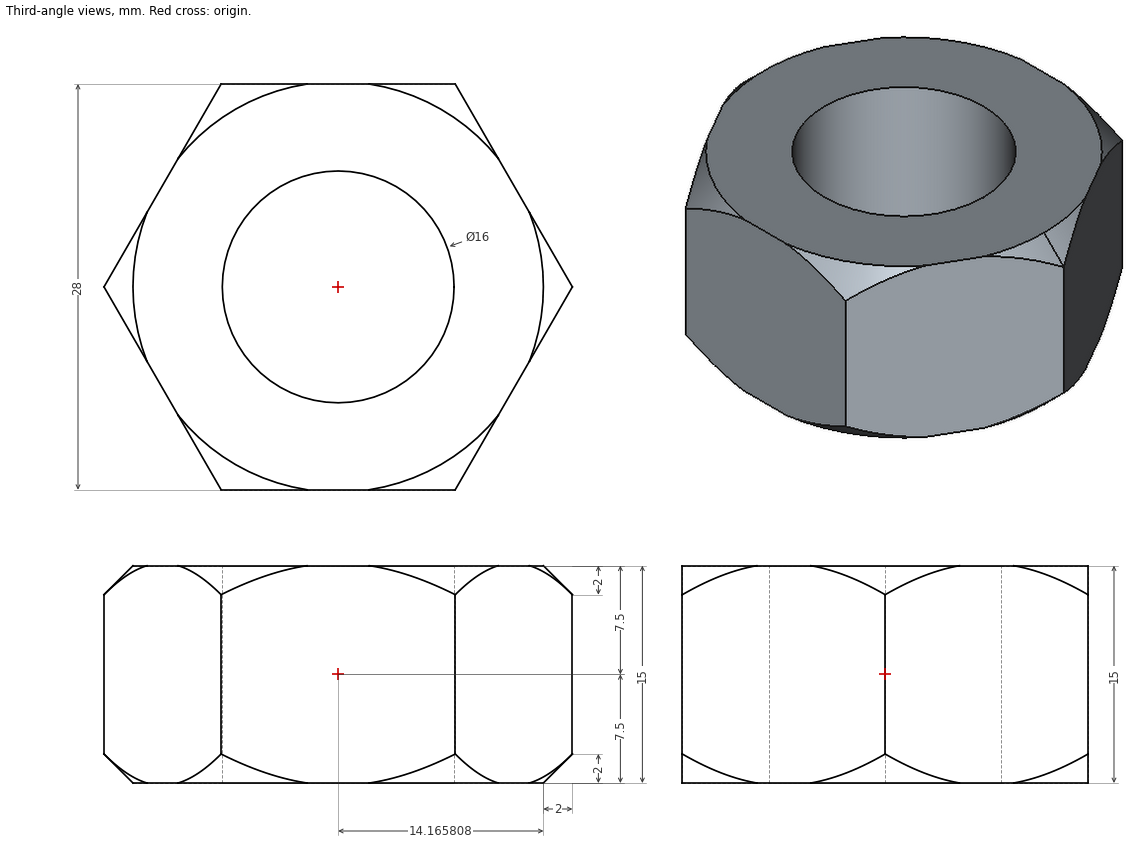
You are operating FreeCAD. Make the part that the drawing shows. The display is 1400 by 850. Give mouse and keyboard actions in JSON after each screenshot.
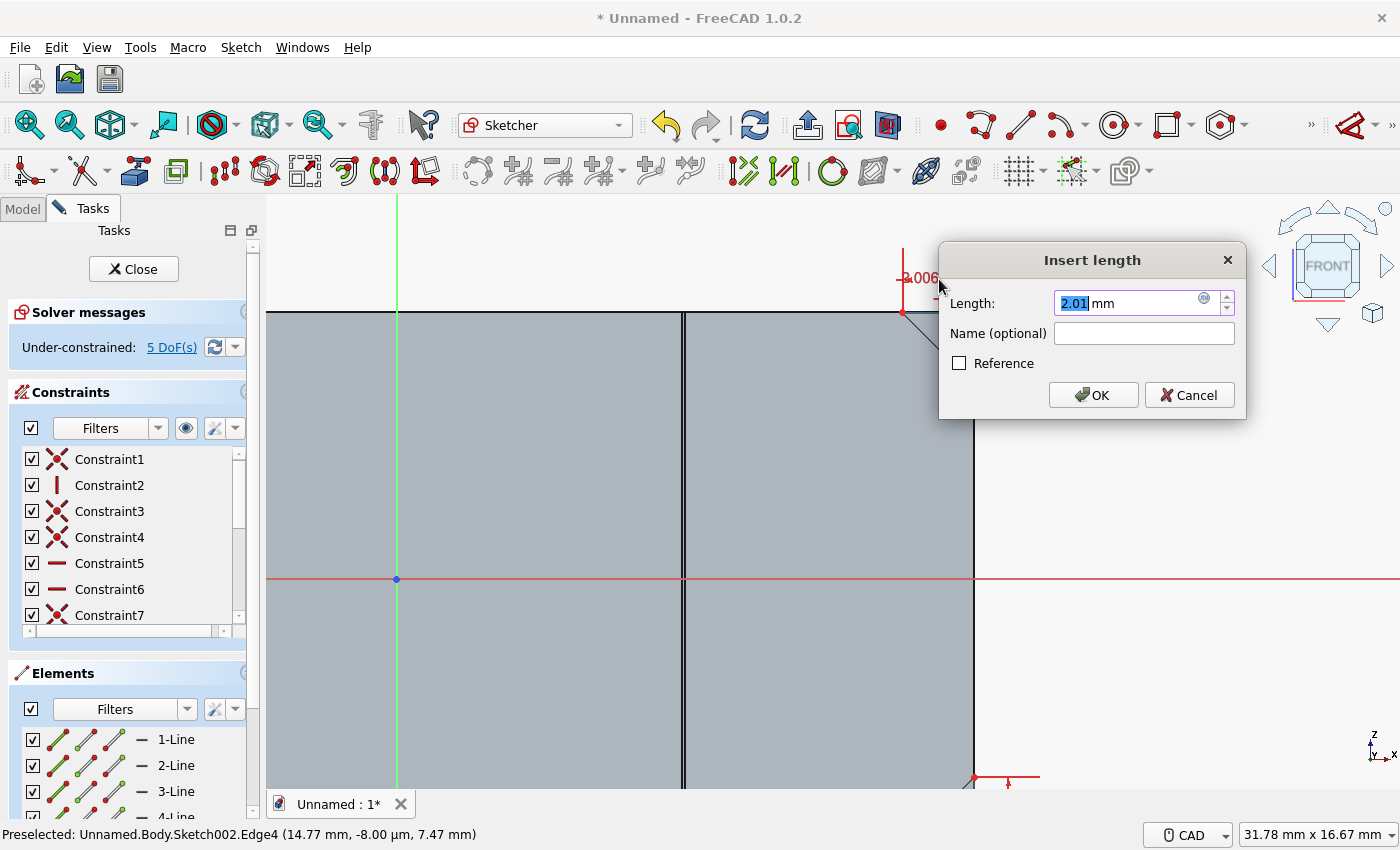
{"action": "type", "text": "2"}
{"action": "key", "text": "Return"}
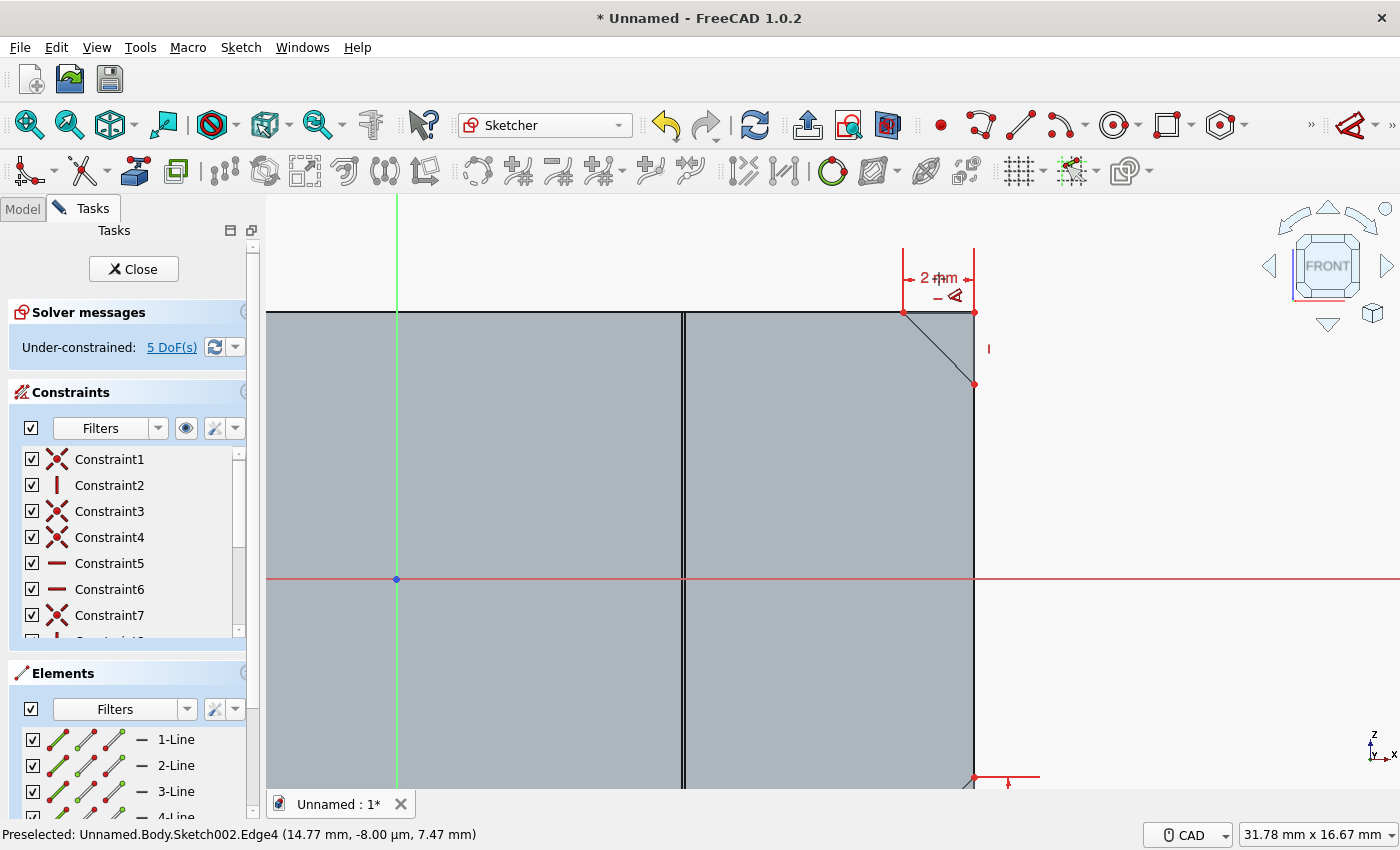
{"action": "left_click", "coordinate": [974, 334]}
{"action": "left_click", "coordinate": [1008, 349]}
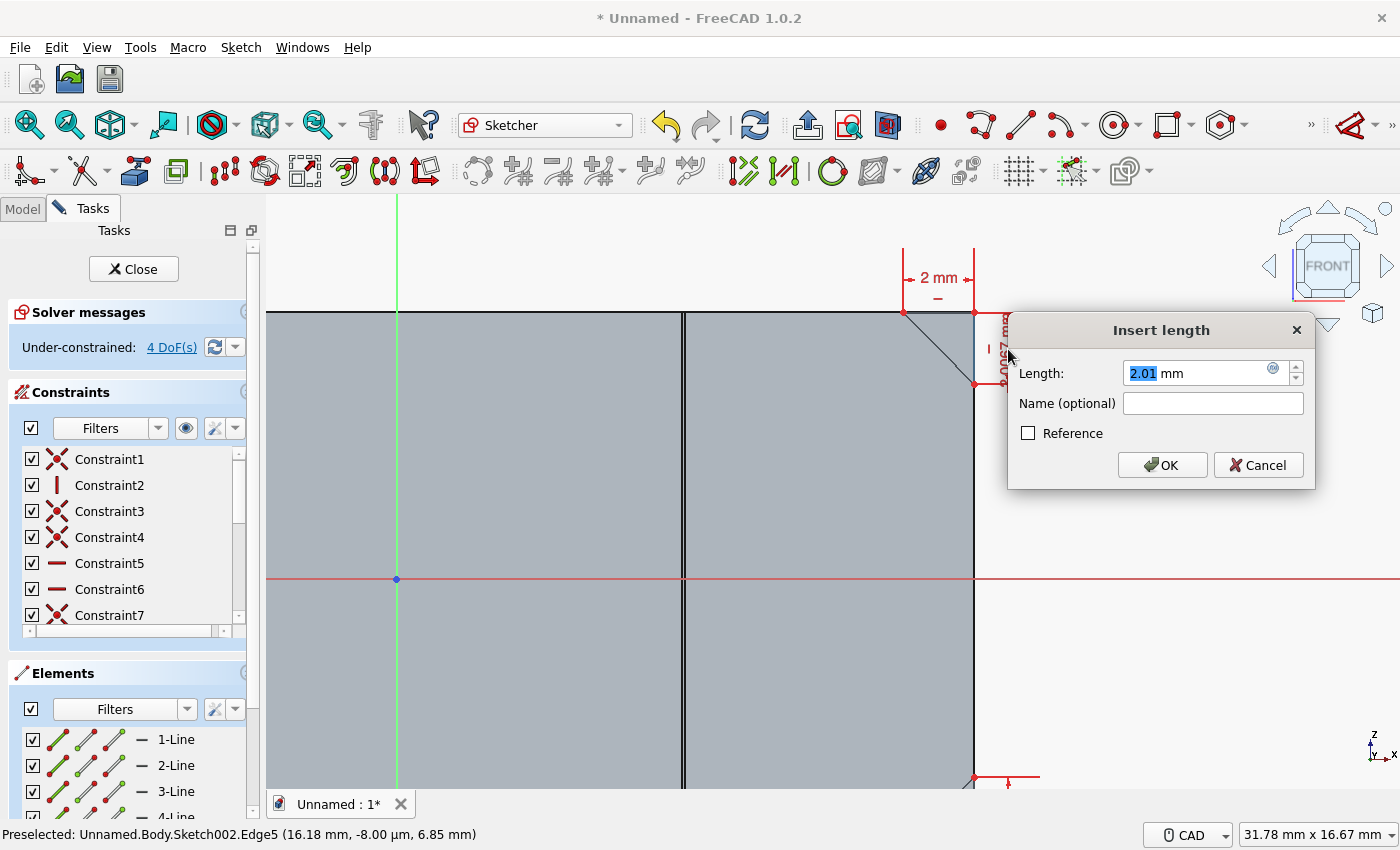
{"action": "type", "text": "2"}
{"action": "key", "text": "Return"}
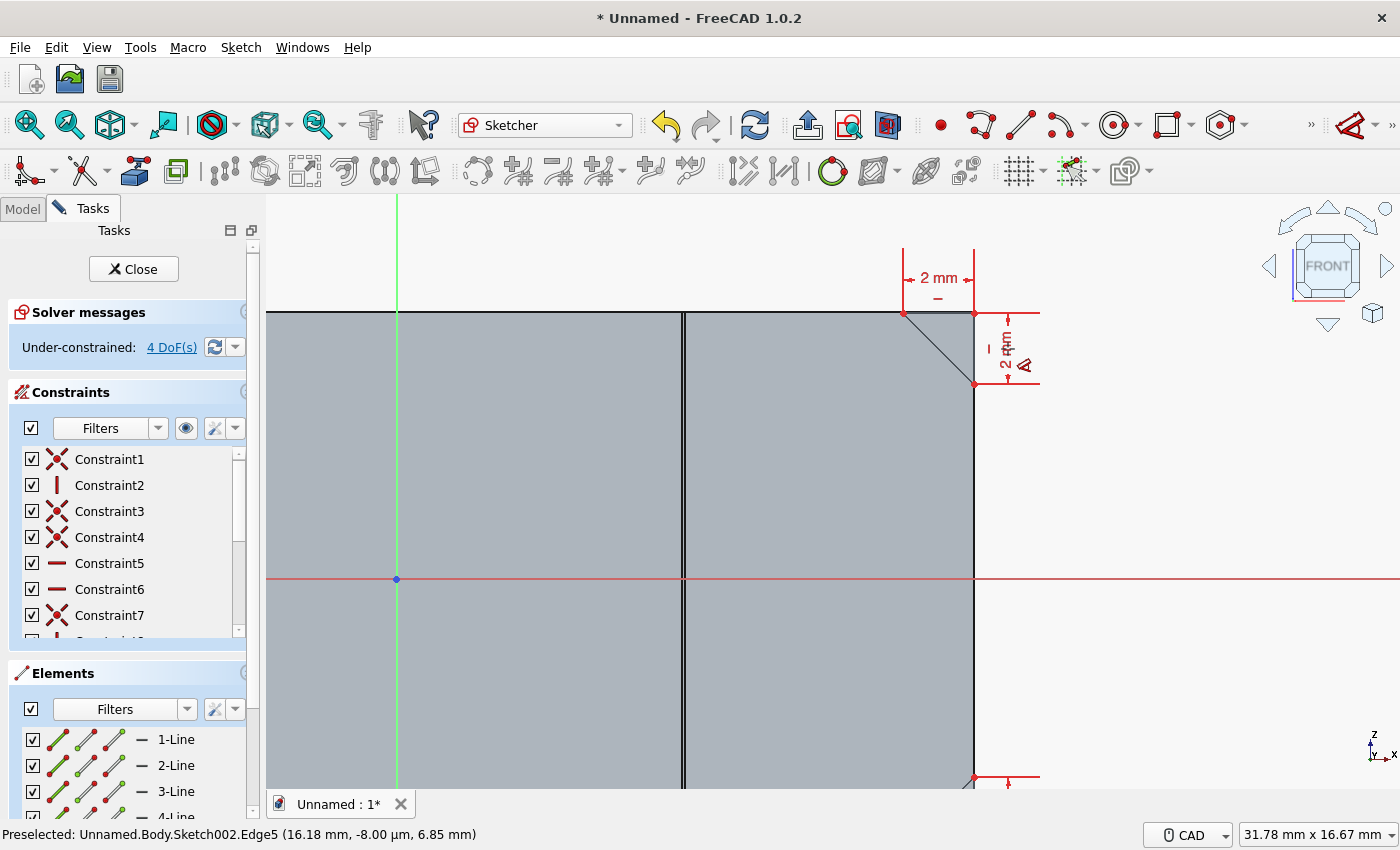
{"action": "scroll", "coordinate": [925, 313], "scroll_direction": "down", "scroll_amount": 2}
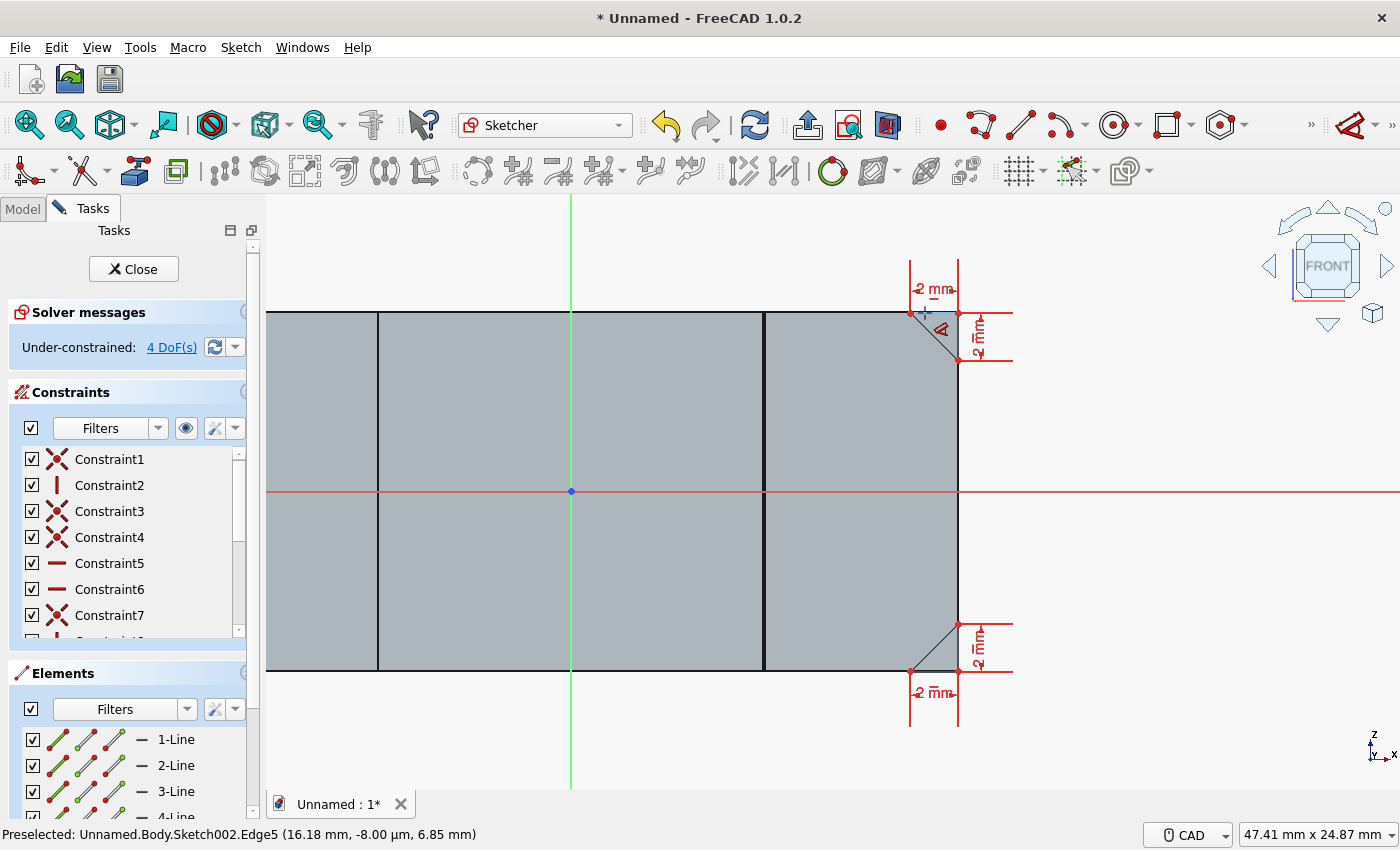
{"action": "left_click", "coordinate": [910, 672]}
{"action": "left_click", "coordinate": [537, 582]}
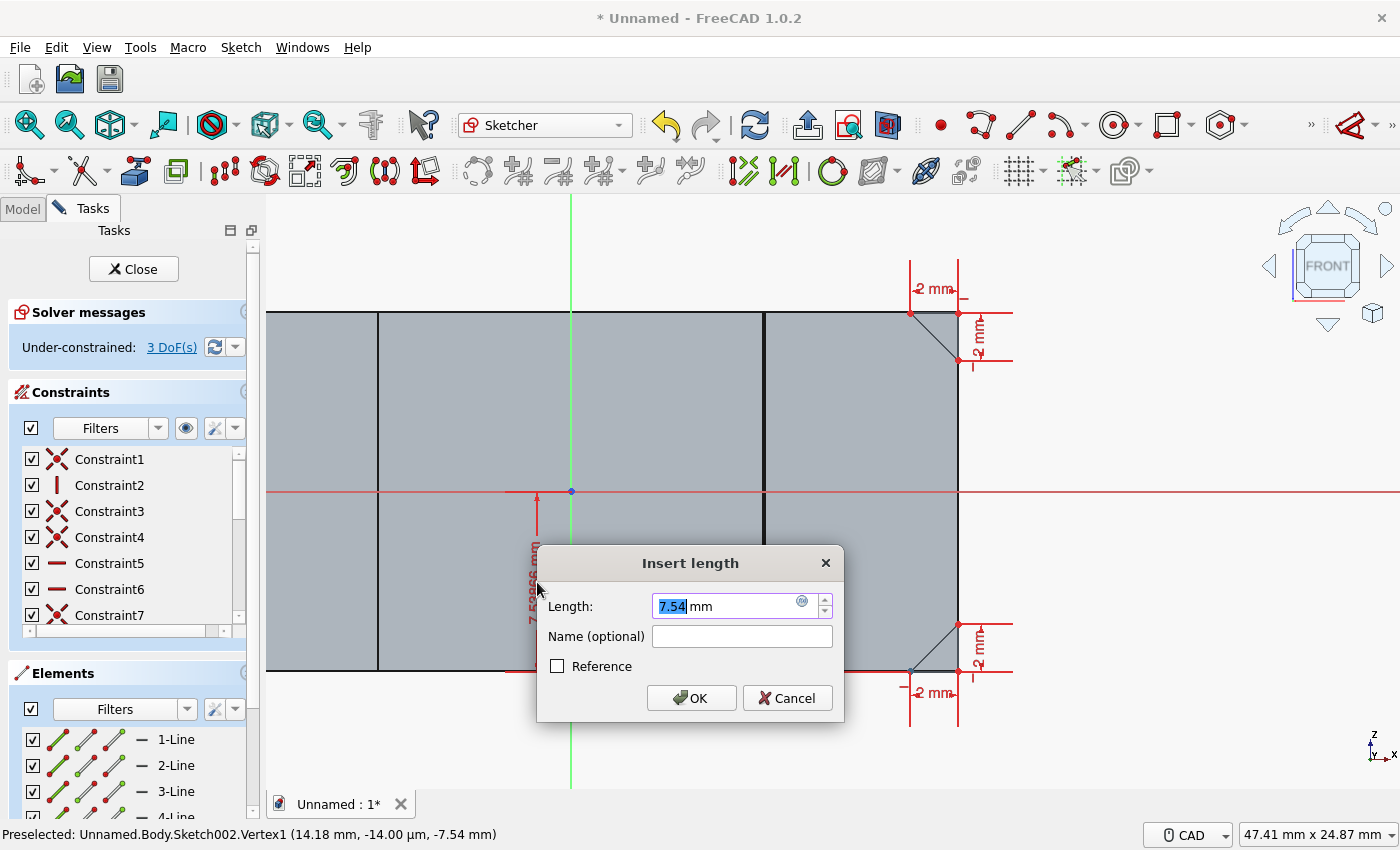
{"action": "type", "text": "7.5"}
{"action": "key", "text": "Return"}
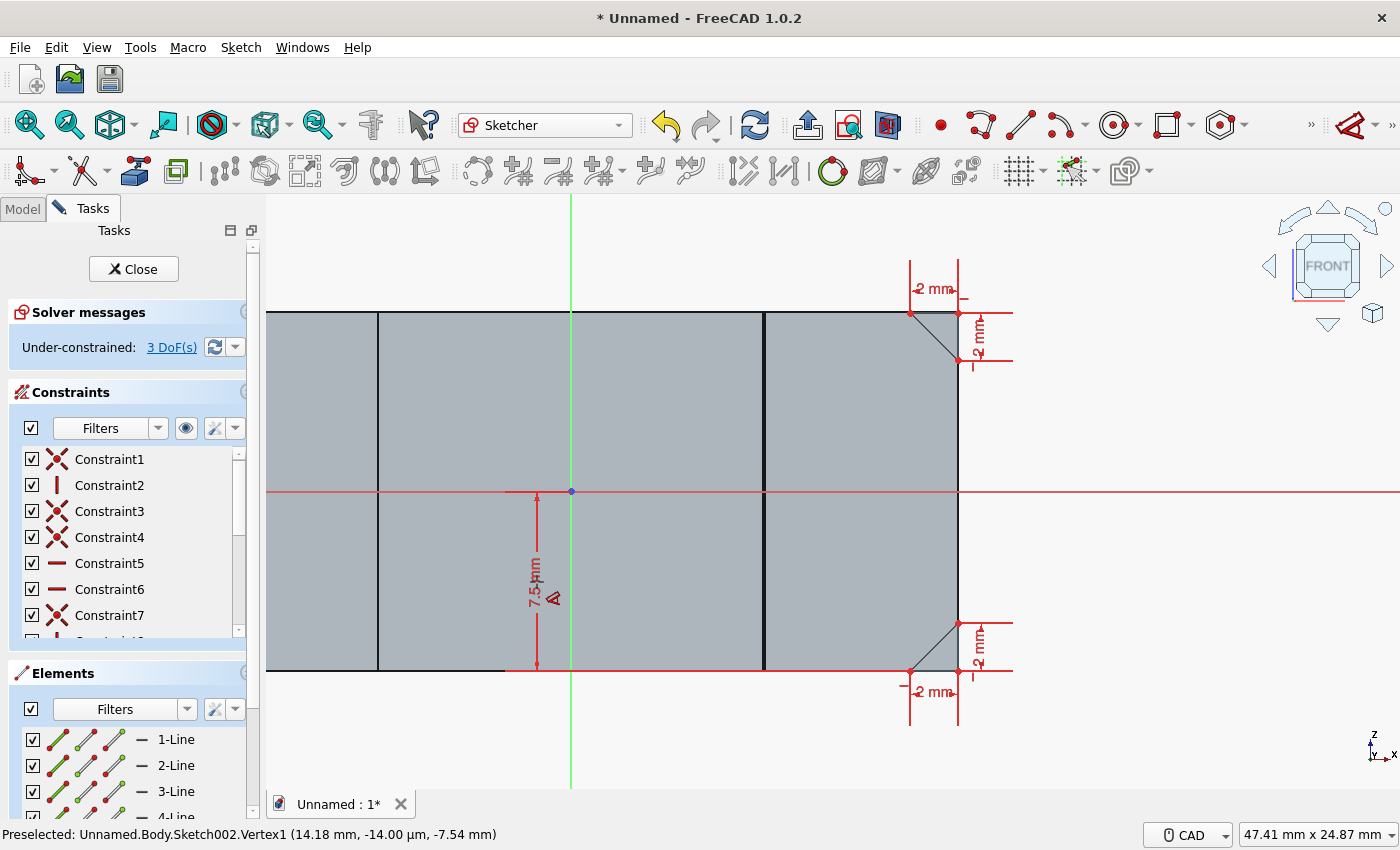
{"action": "left_click", "coordinate": [910, 313]}
{"action": "left_click", "coordinate": [537, 402]}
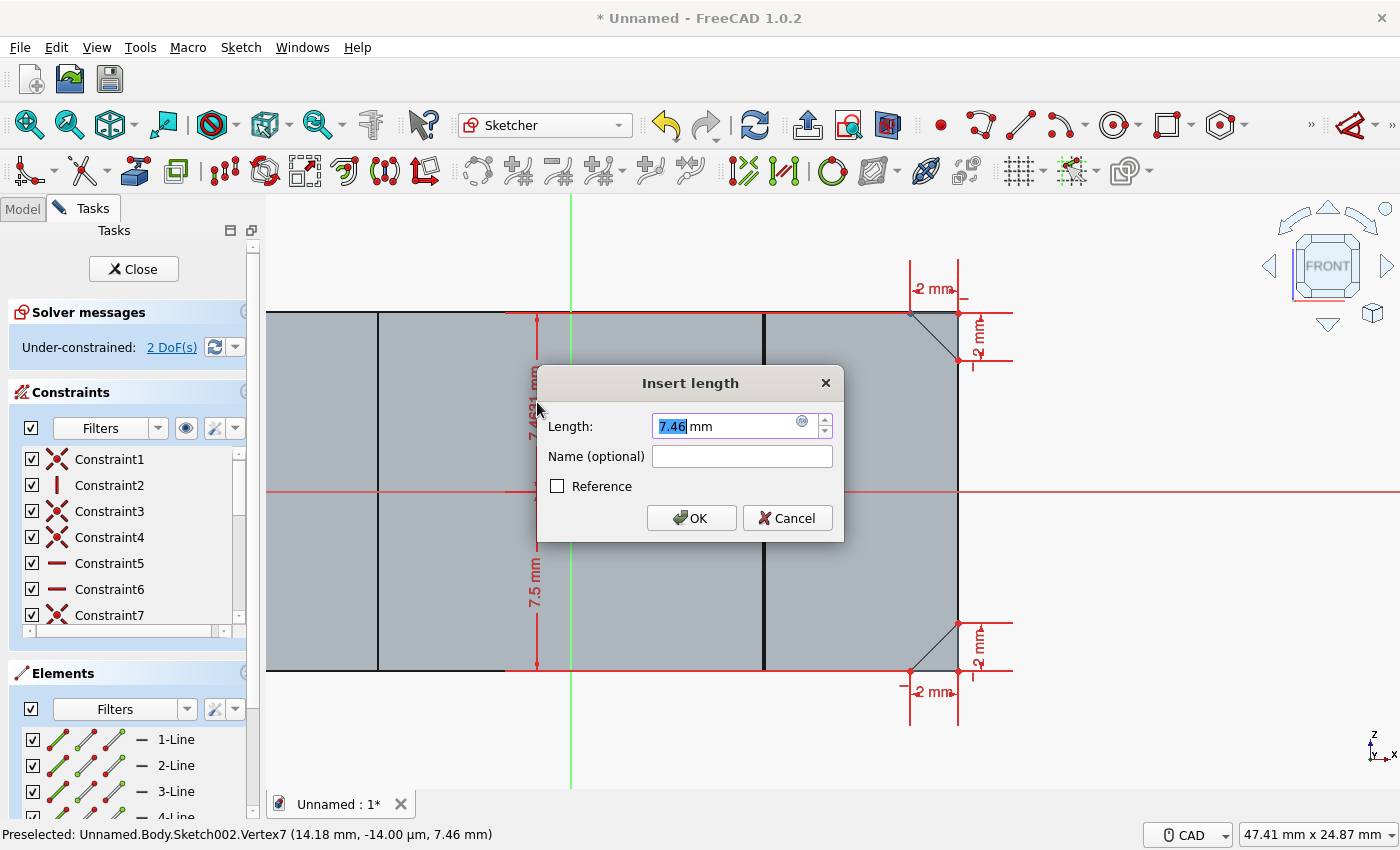
{"action": "type", "text": "7.5"}
{"action": "key", "text": "Return"}